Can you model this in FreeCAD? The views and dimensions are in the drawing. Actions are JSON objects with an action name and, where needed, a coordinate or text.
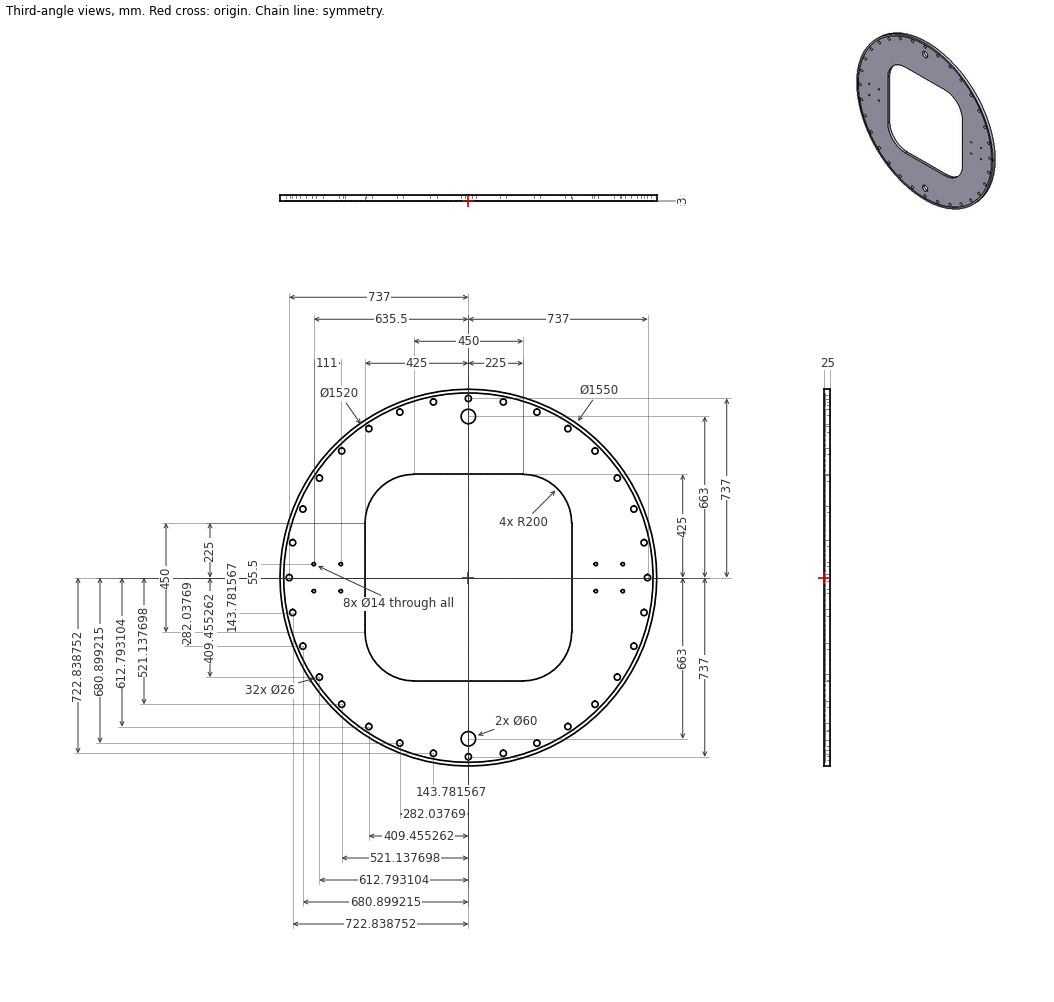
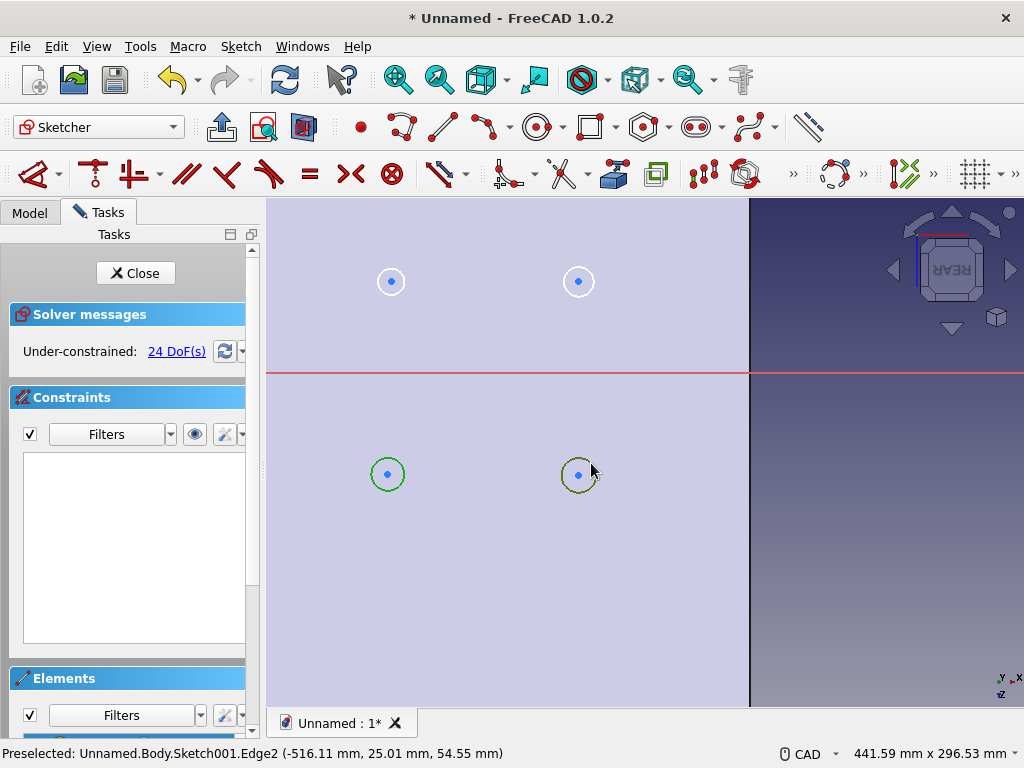
{"action": "left_click", "coordinate": [589, 271]}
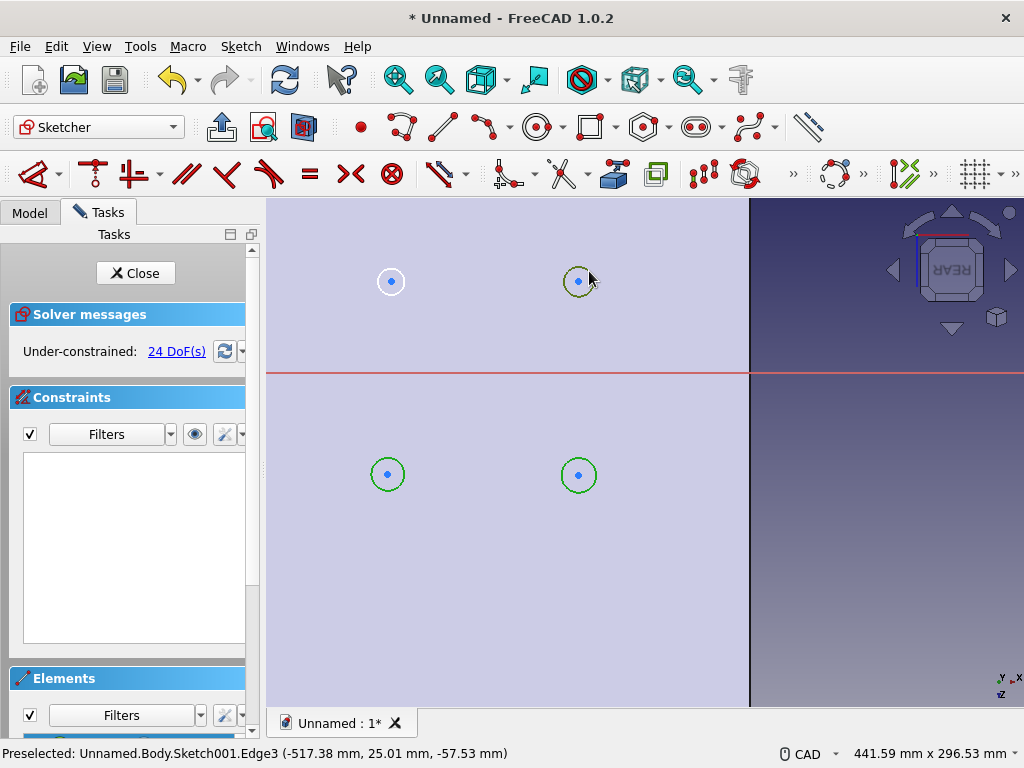
{"action": "left_click", "coordinate": [401, 272]}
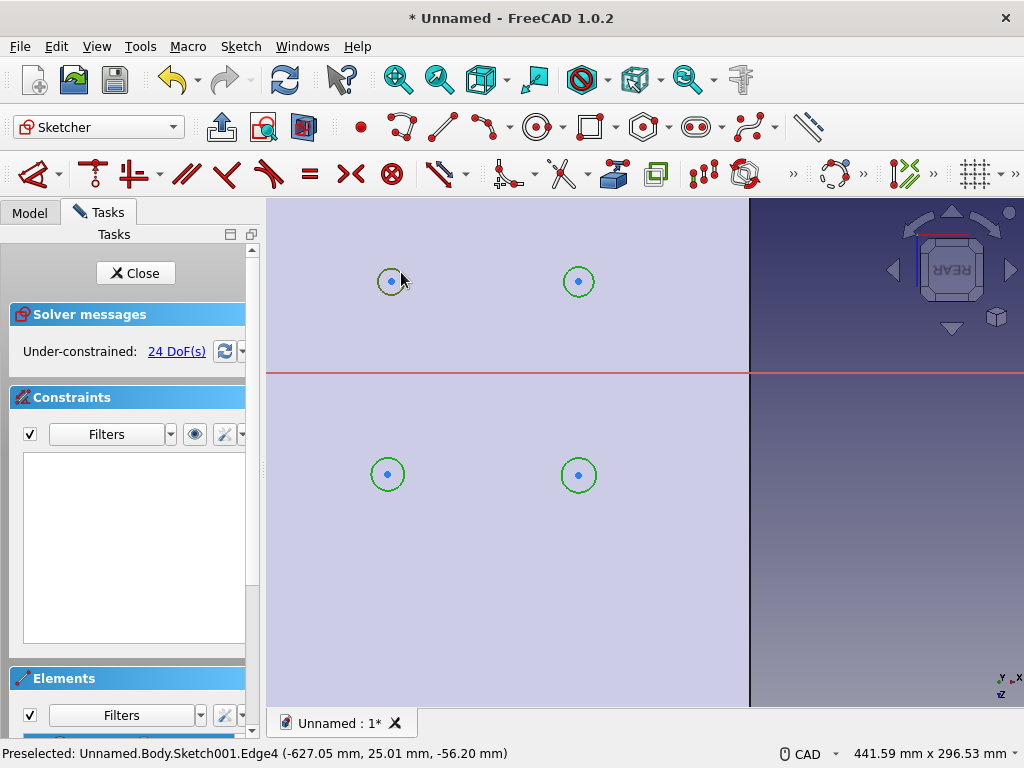
{"action": "scroll", "coordinate": [398, 468], "scroll_direction": "down", "scroll_amount": 9}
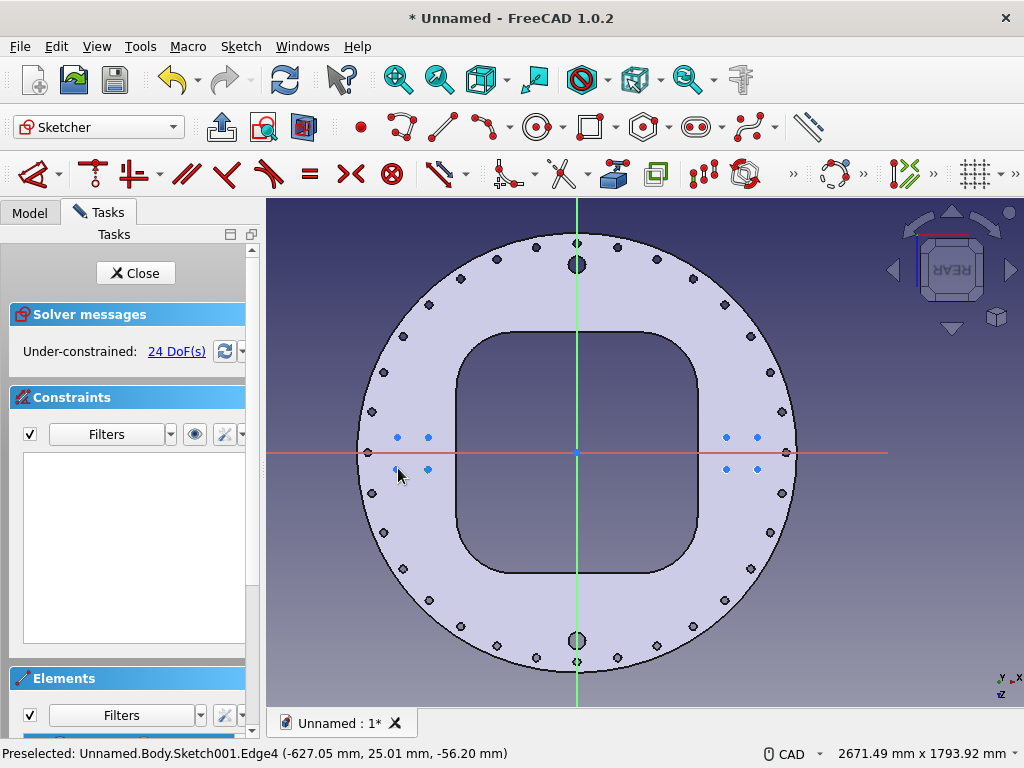
{"action": "scroll", "coordinate": [759, 436], "scroll_direction": "up", "scroll_amount": 9}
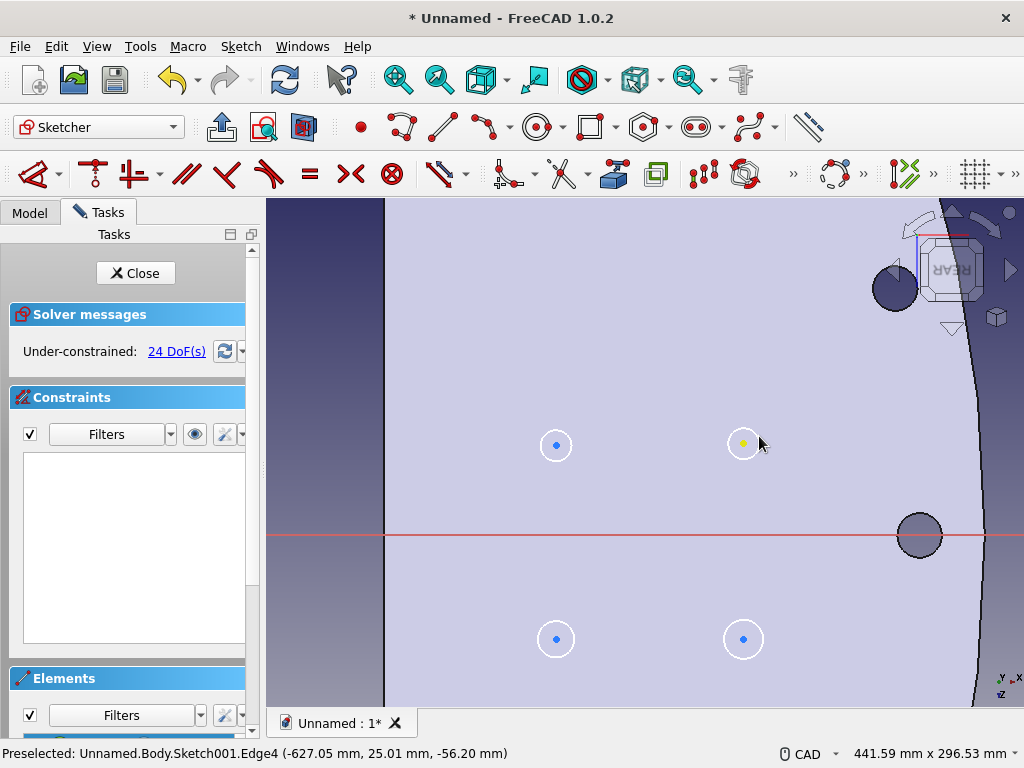
{"action": "left_click", "coordinate": [755, 433]}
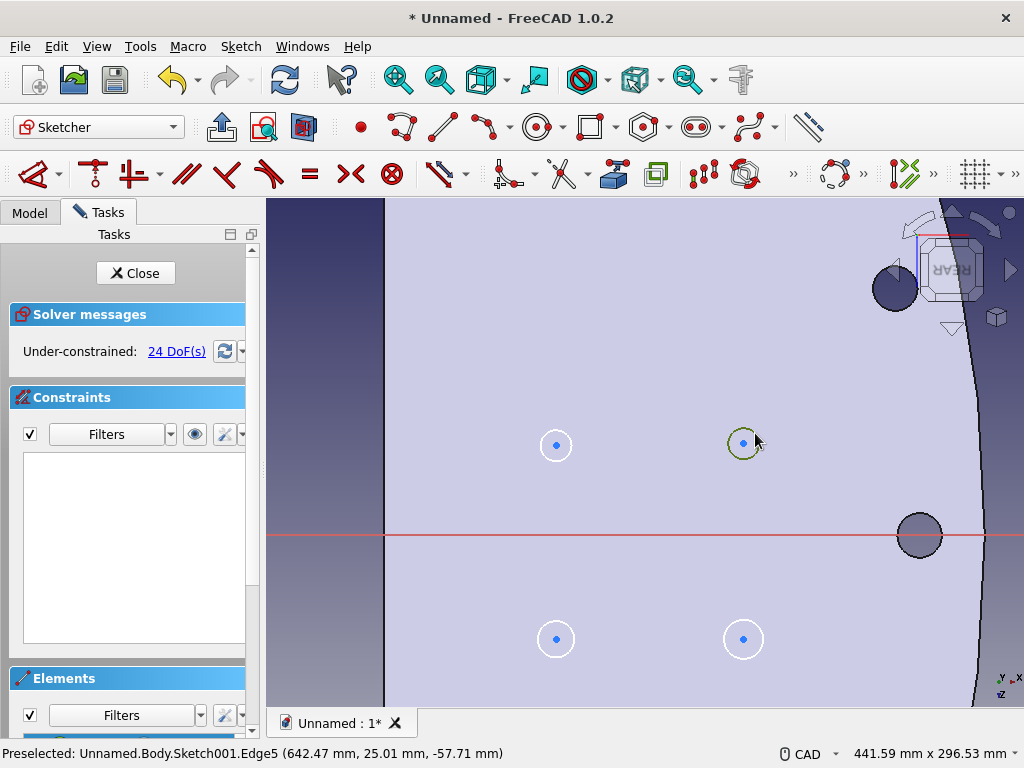
{"action": "left_click", "coordinate": [567, 435]}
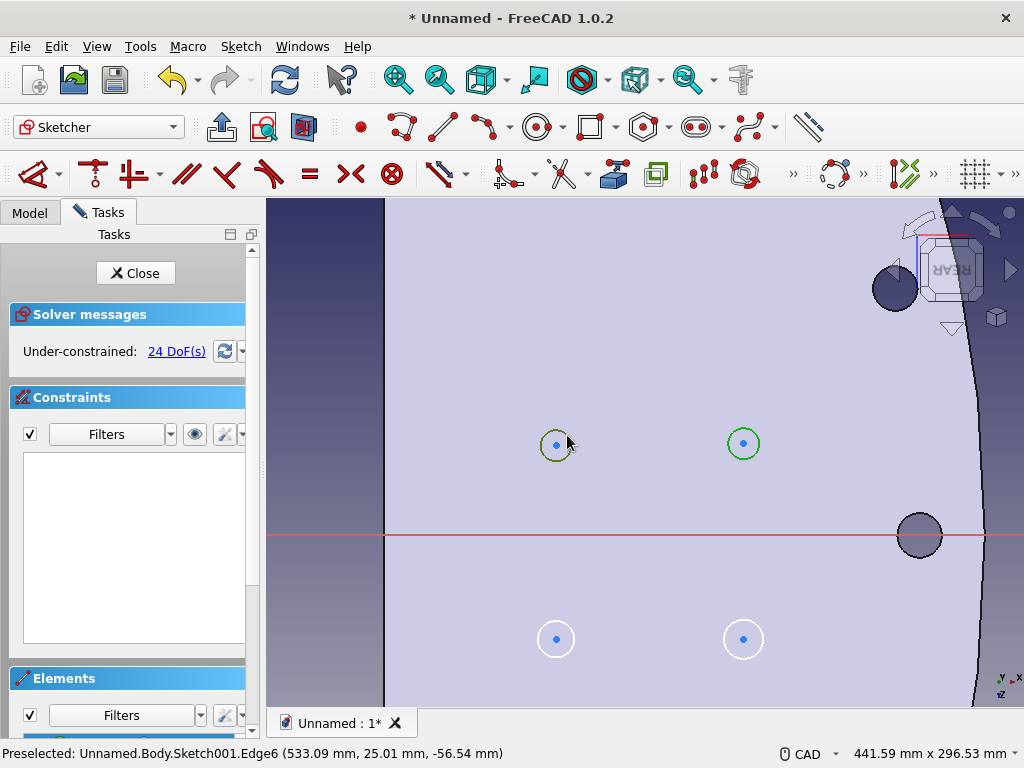
{"action": "left_click", "coordinate": [569, 626]}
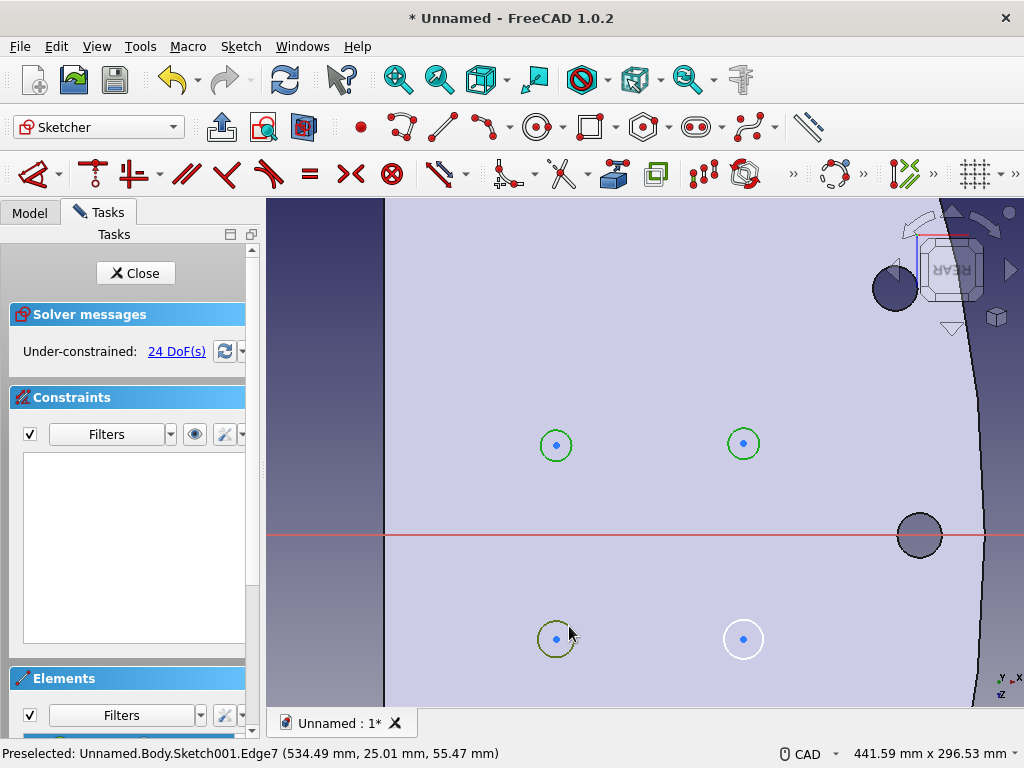
{"action": "left_click", "coordinate": [757, 625]}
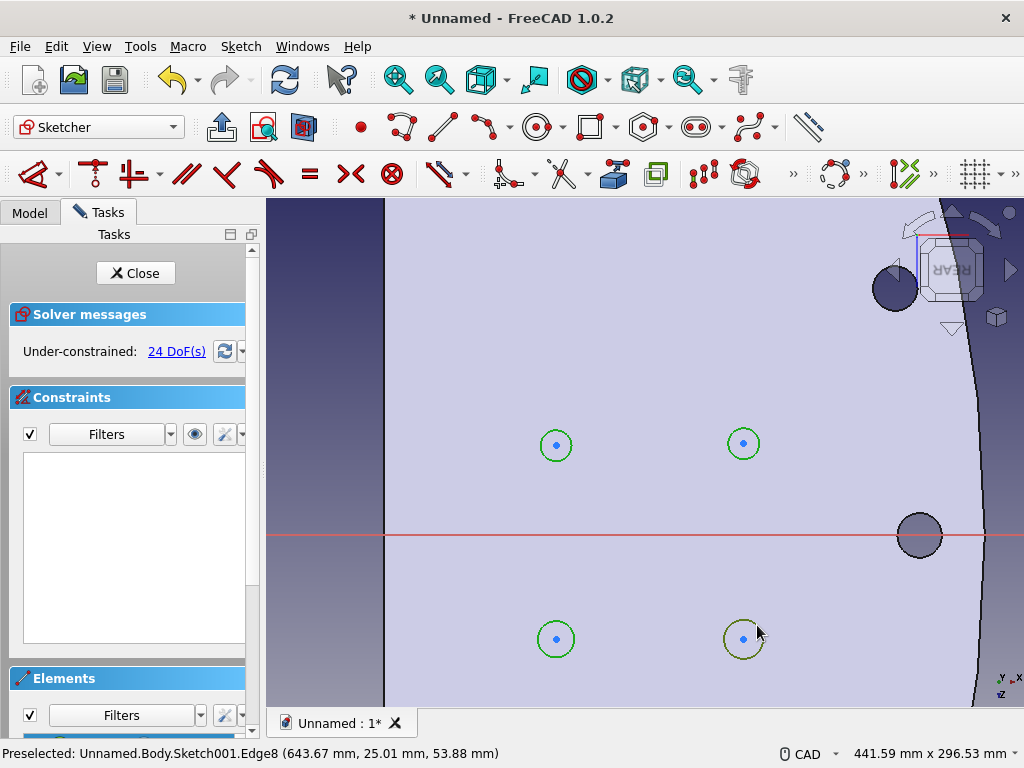
{"action": "left_click", "coordinate": [310, 174]}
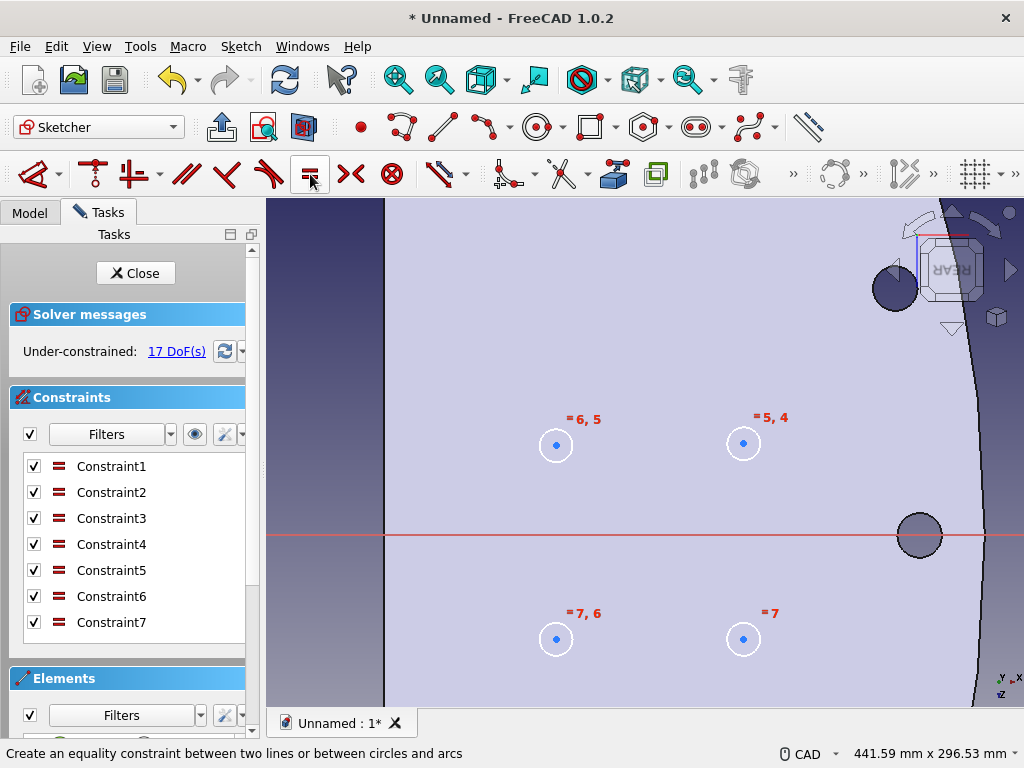
{"action": "scroll", "coordinate": [759, 436], "scroll_direction": "down", "scroll_amount": 9}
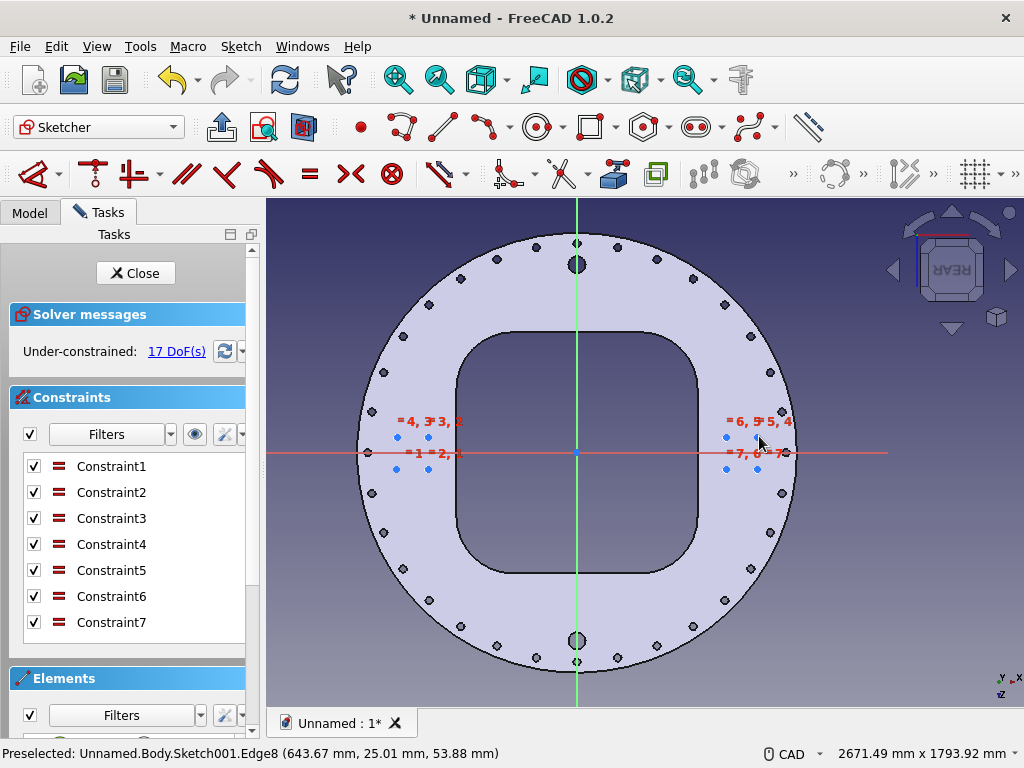
{"action": "left_click", "coordinate": [428, 470]}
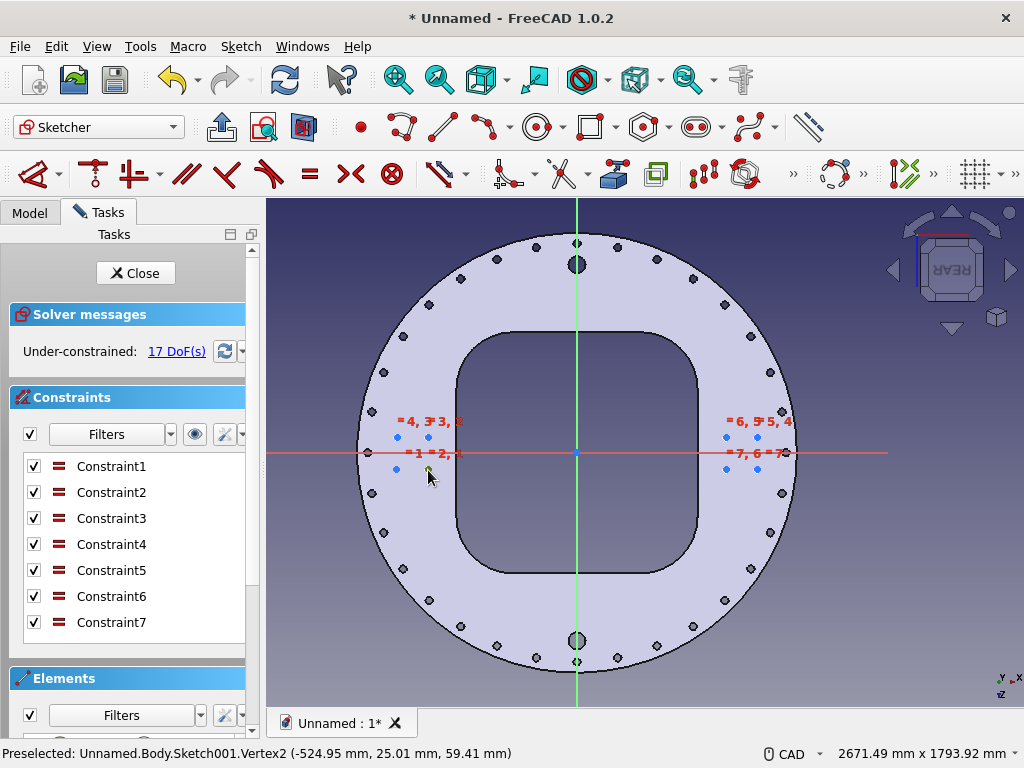
{"action": "left_click", "coordinate": [428, 438]}